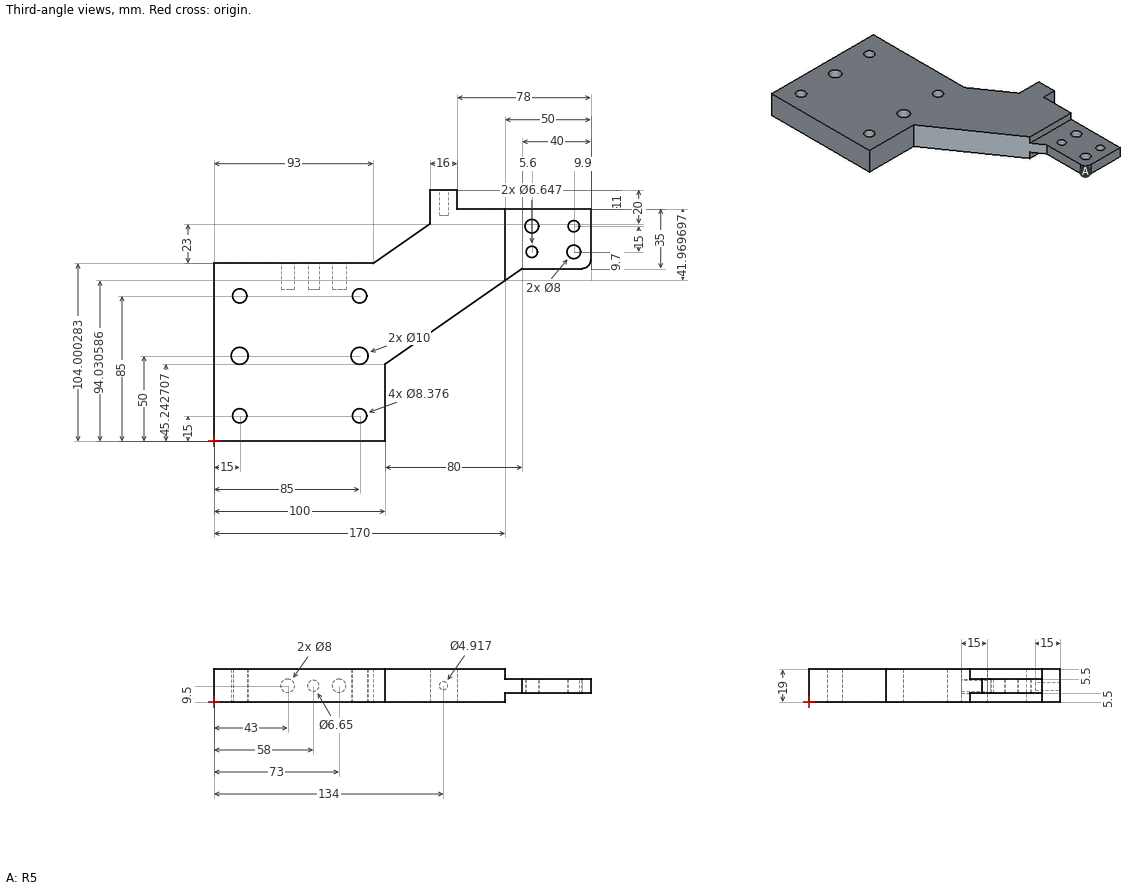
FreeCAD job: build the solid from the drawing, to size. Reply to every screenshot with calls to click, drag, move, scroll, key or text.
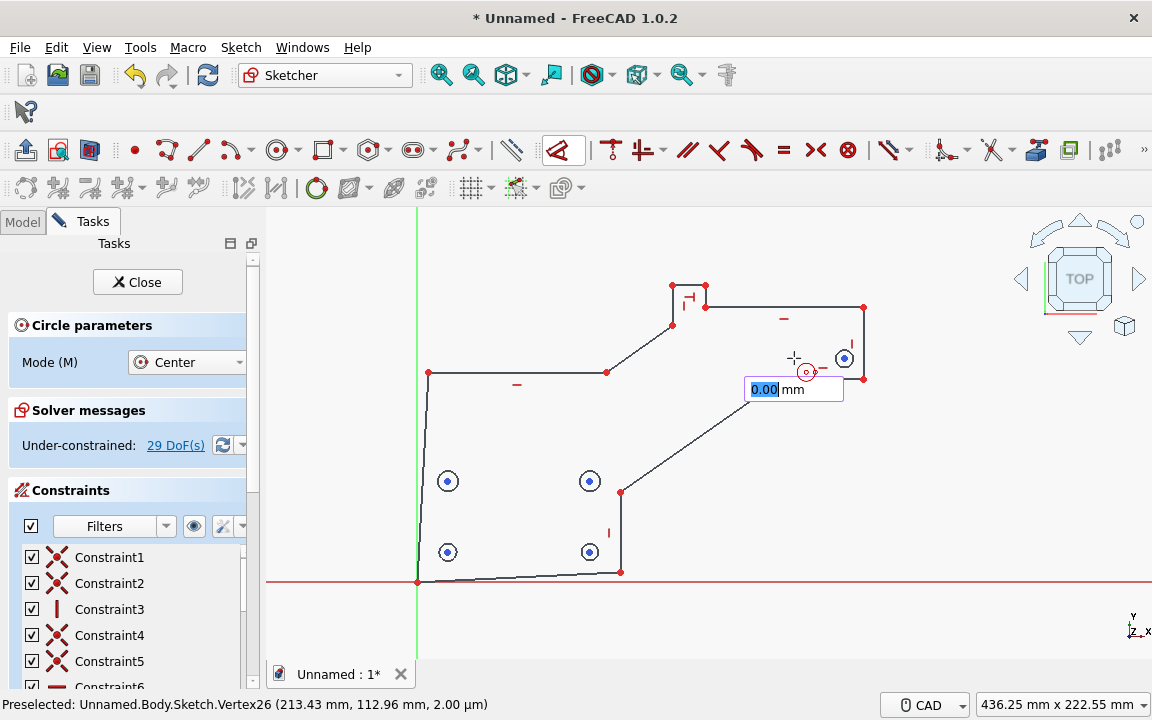
scroll(799, 353, up, 5)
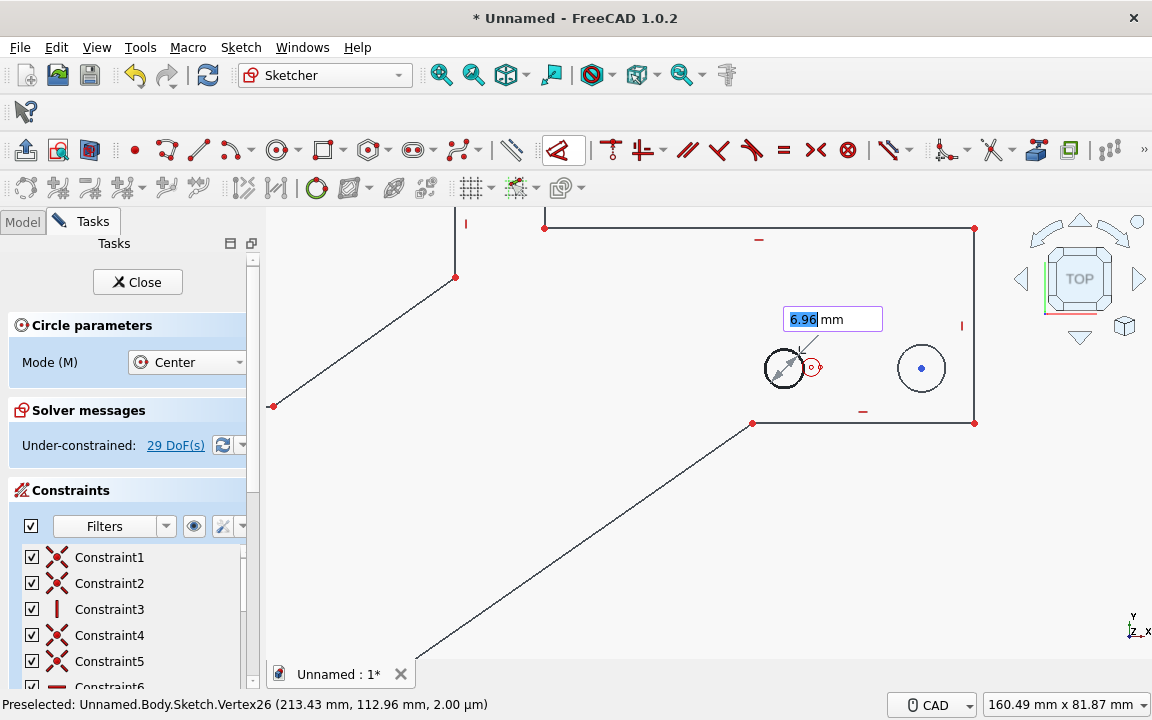
click(798, 352)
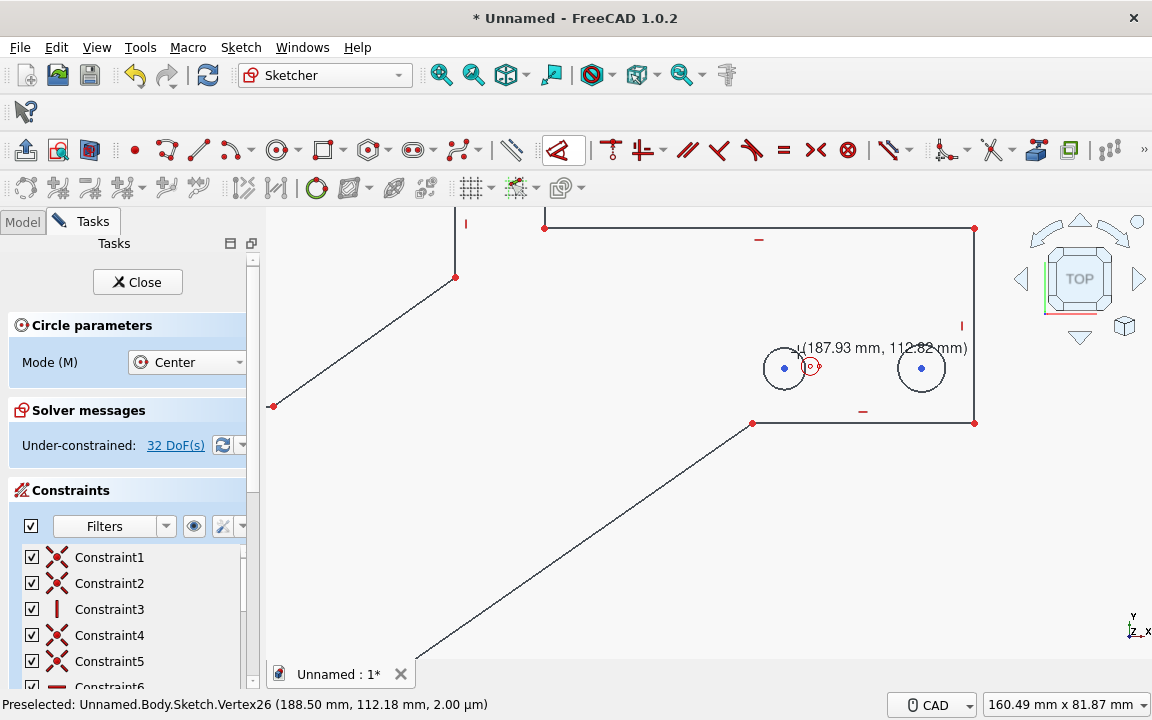
scroll(920, 282, up, 2)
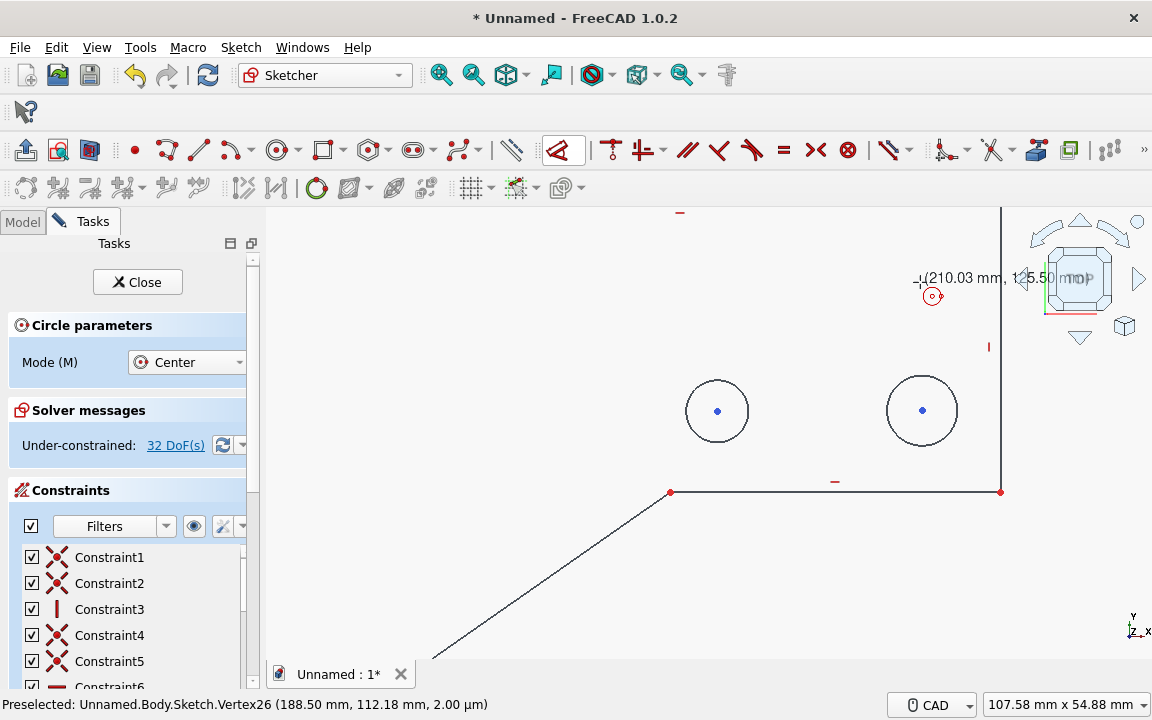
scroll(819, 342, down, 7)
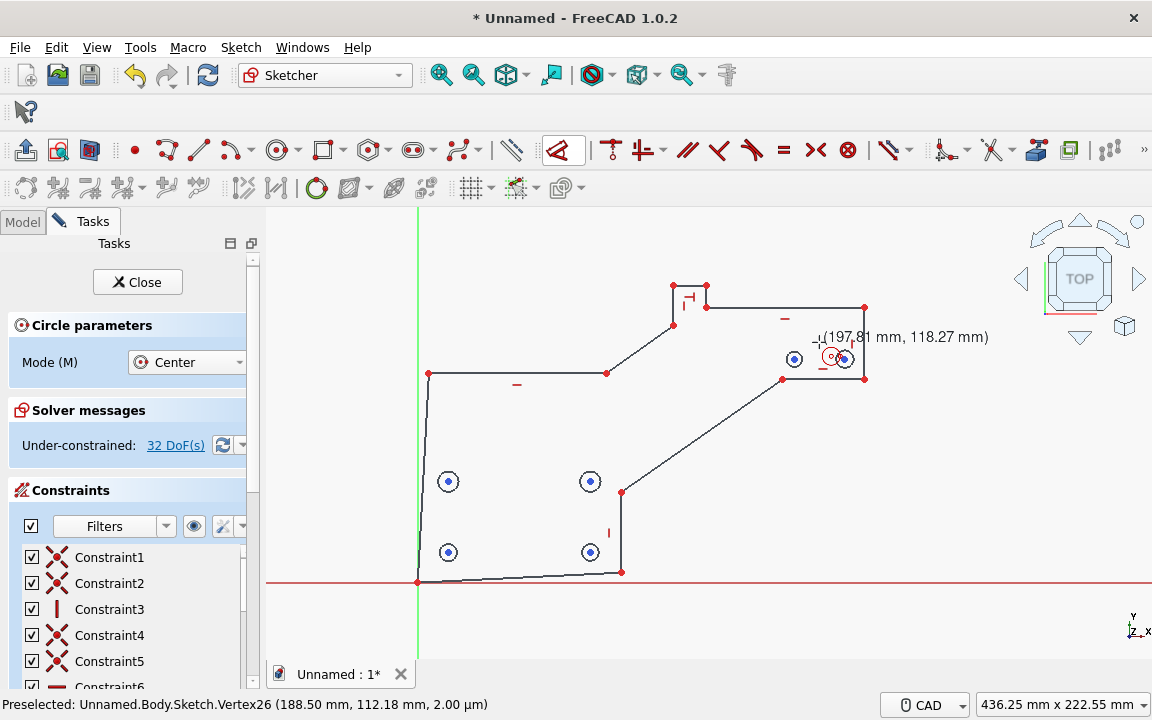
click(844, 327)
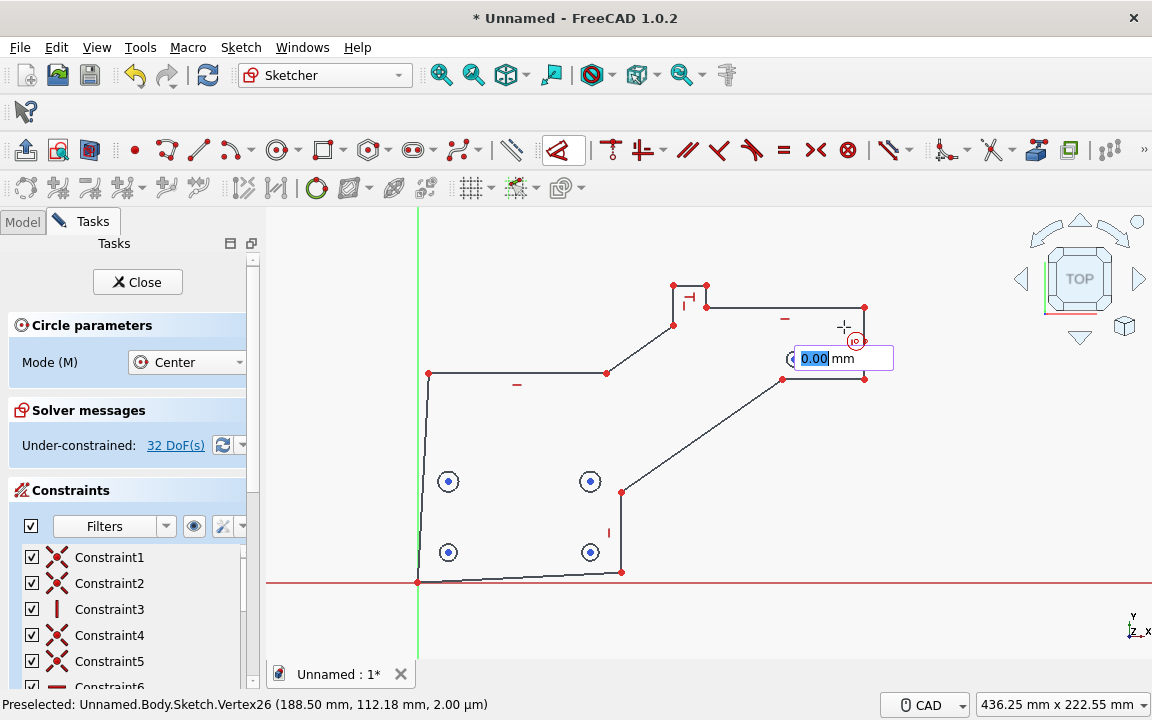
scroll(849, 323, up, 5)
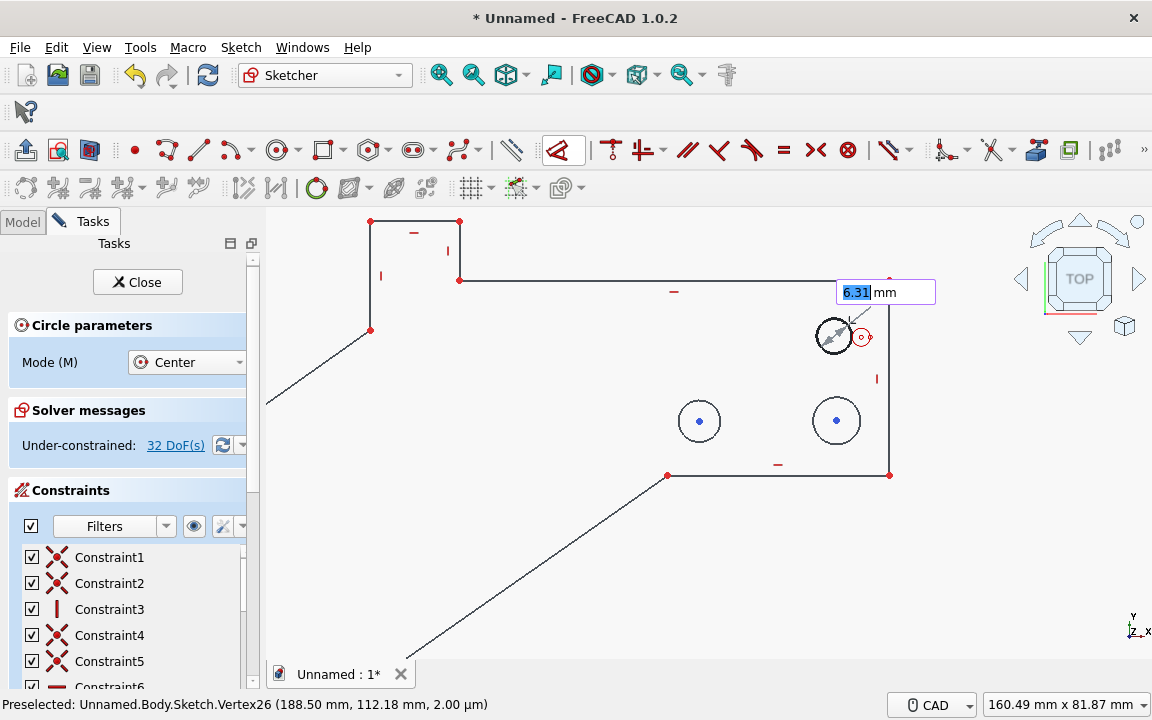
click(848, 321)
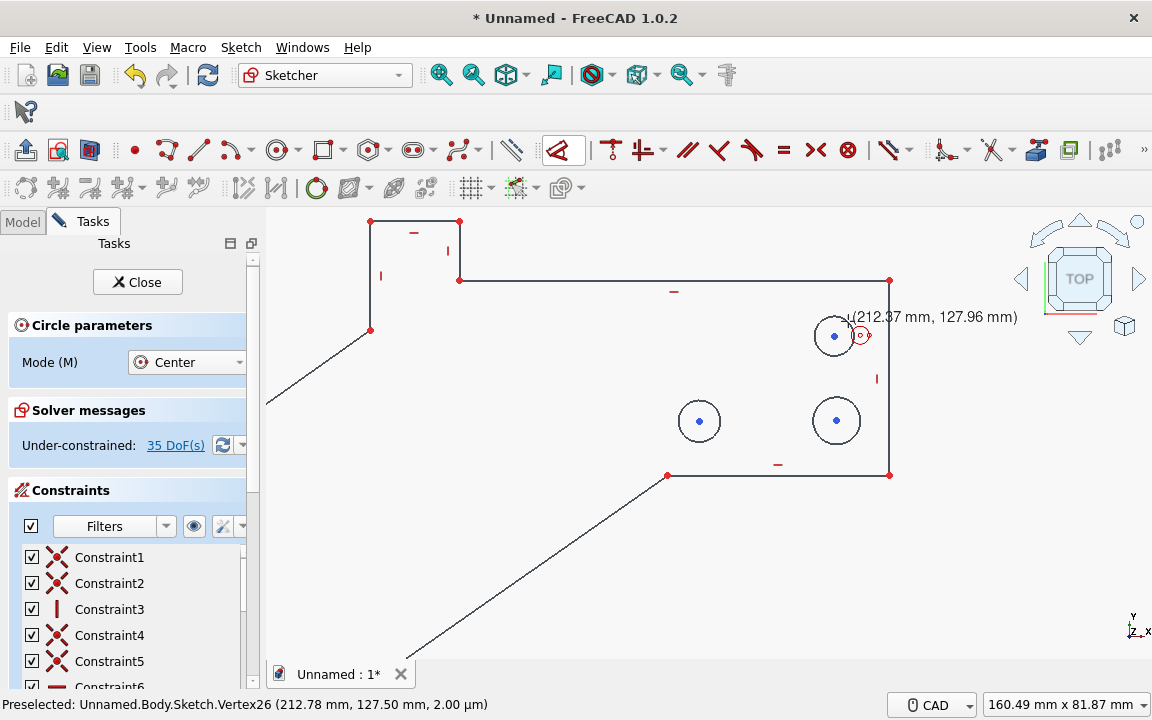
click(700, 334)
click(716, 319)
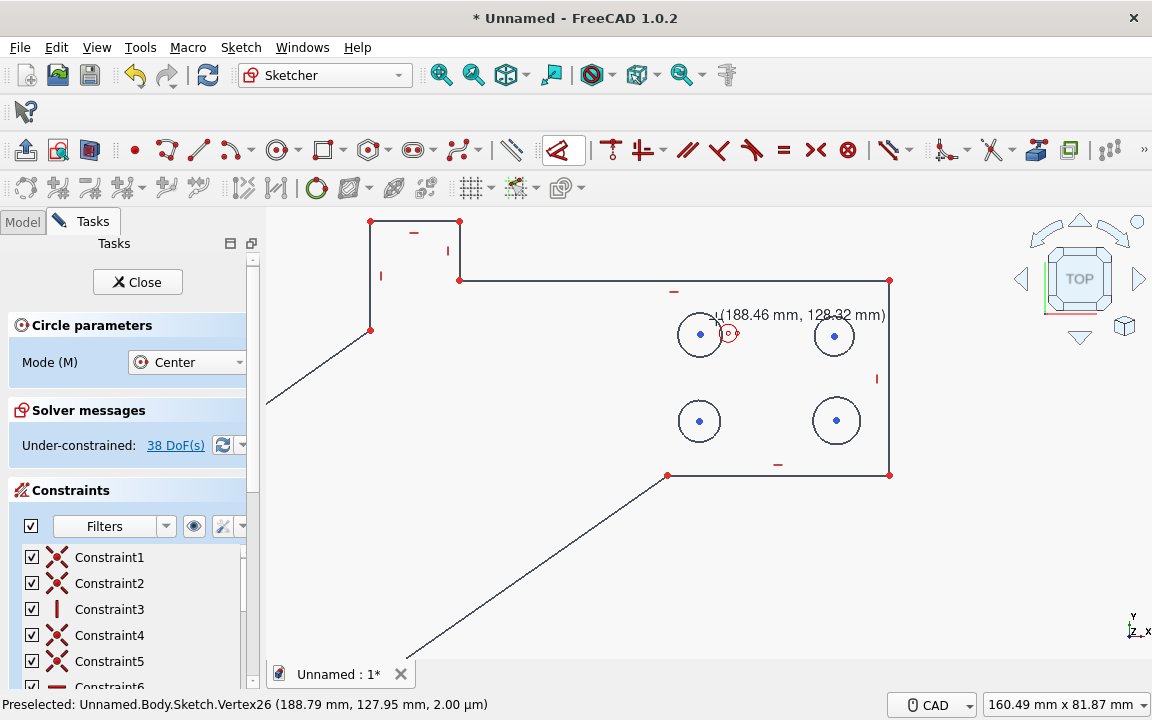
scroll(849, 323, down, 5)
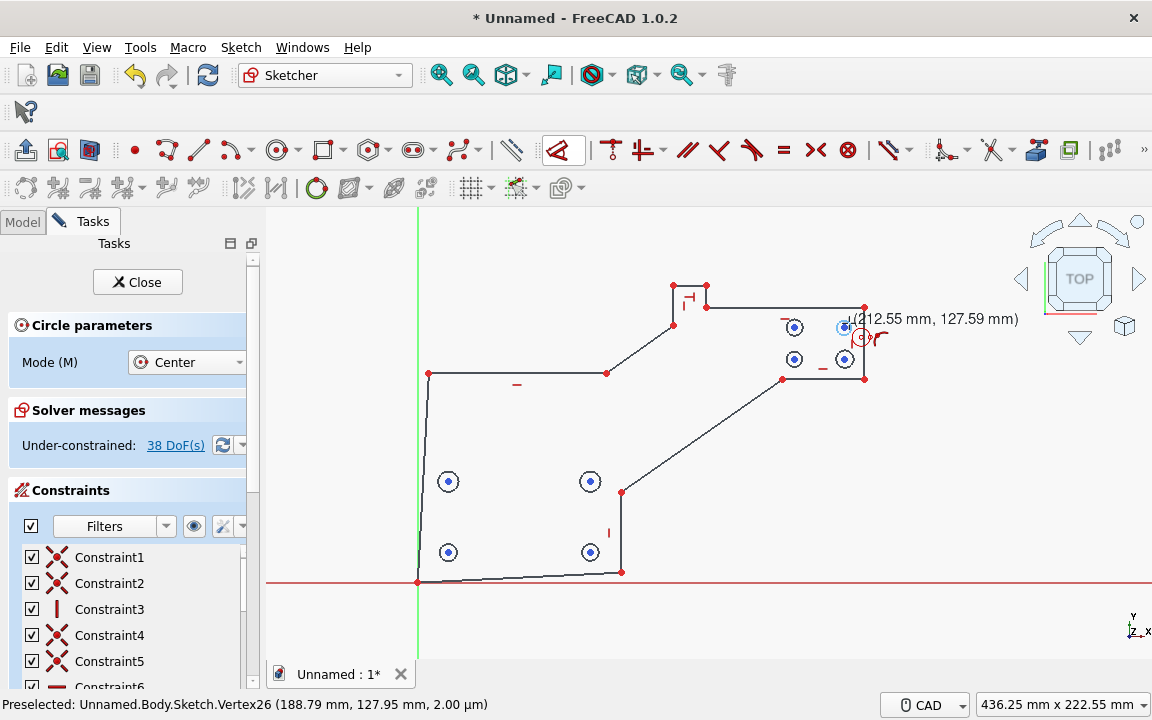
scroll(590, 410, up, 5)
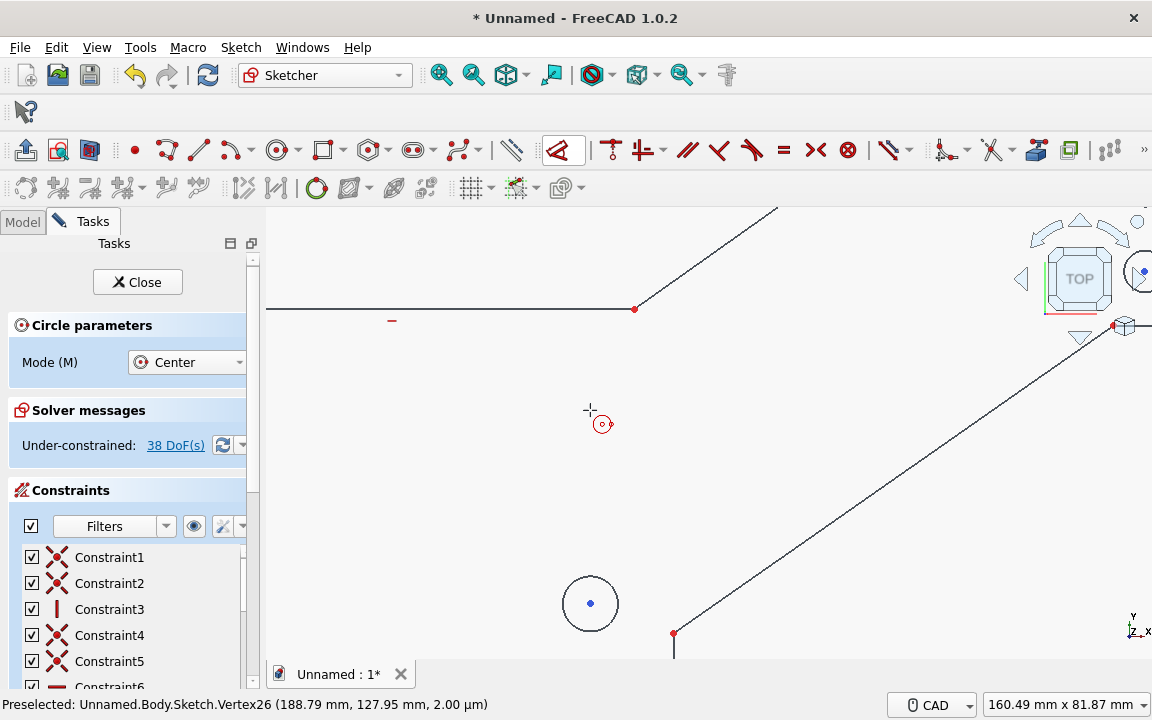
click(590, 409)
click(607, 393)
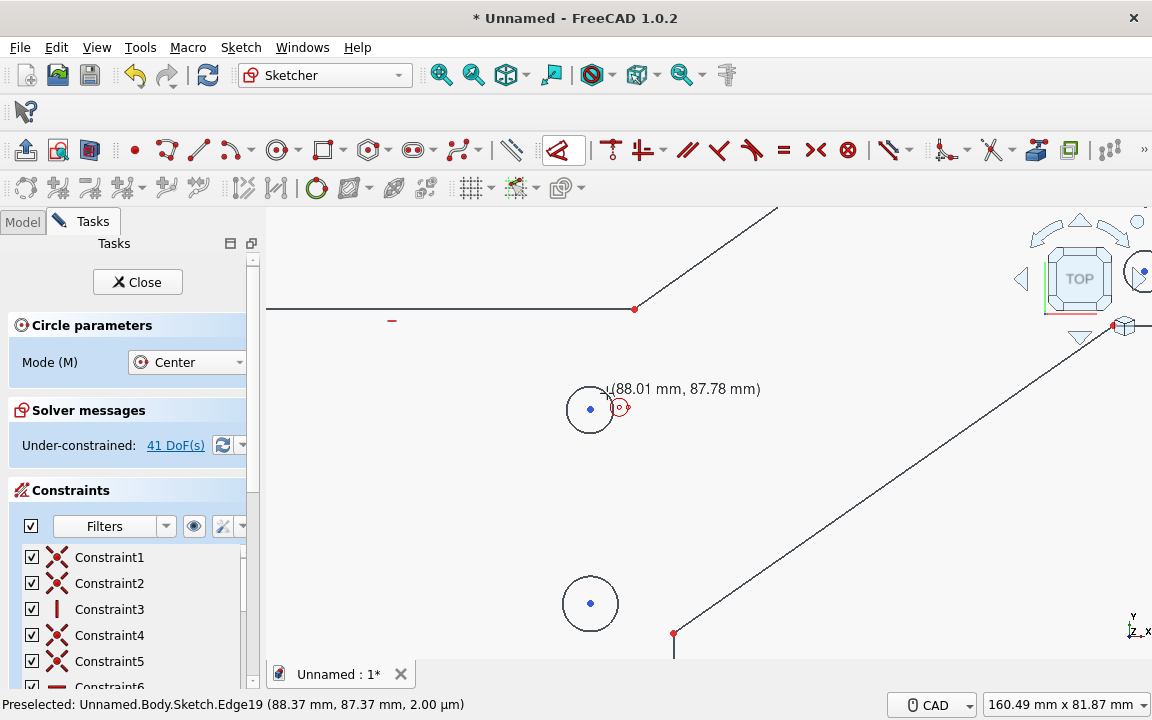
scroll(589, 410, down, 5)